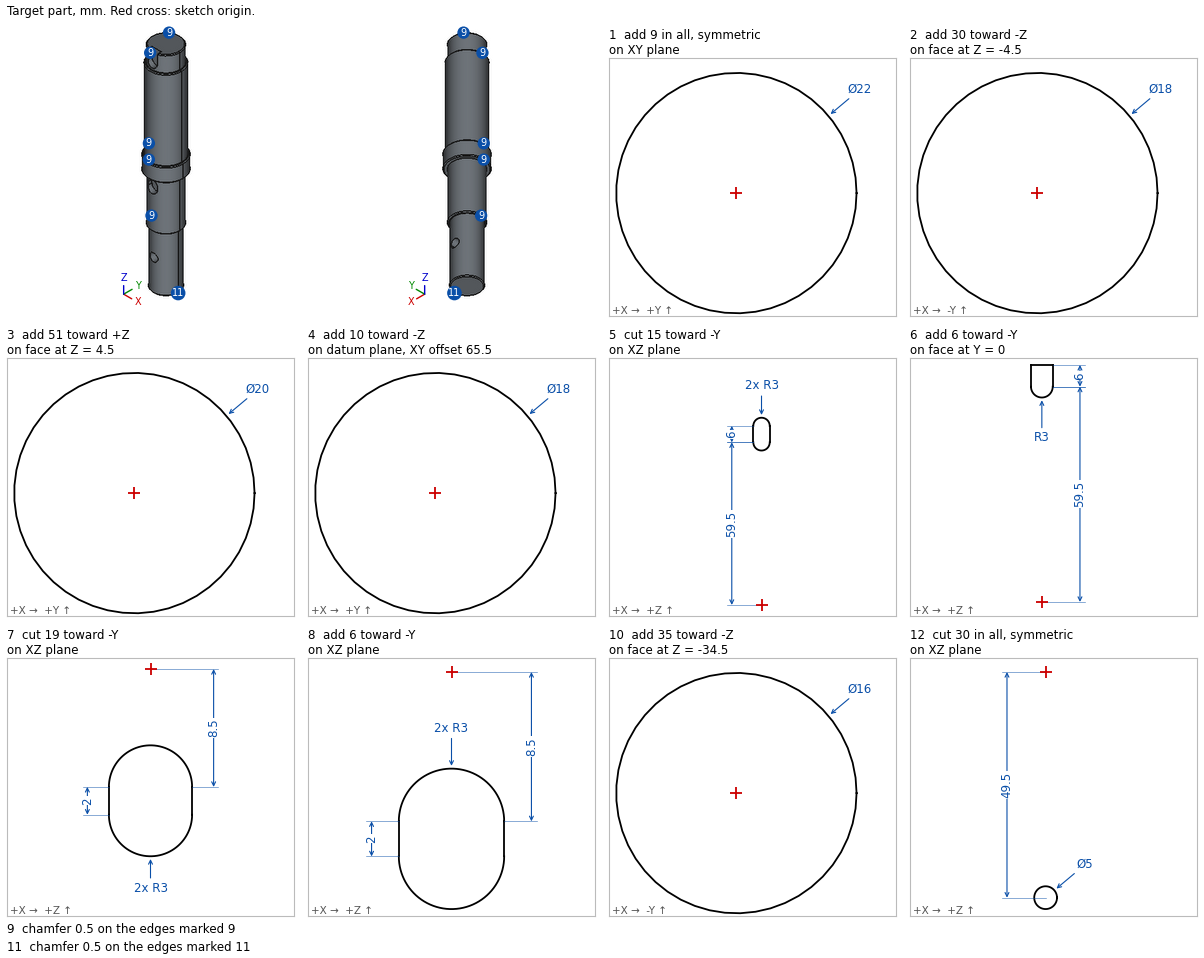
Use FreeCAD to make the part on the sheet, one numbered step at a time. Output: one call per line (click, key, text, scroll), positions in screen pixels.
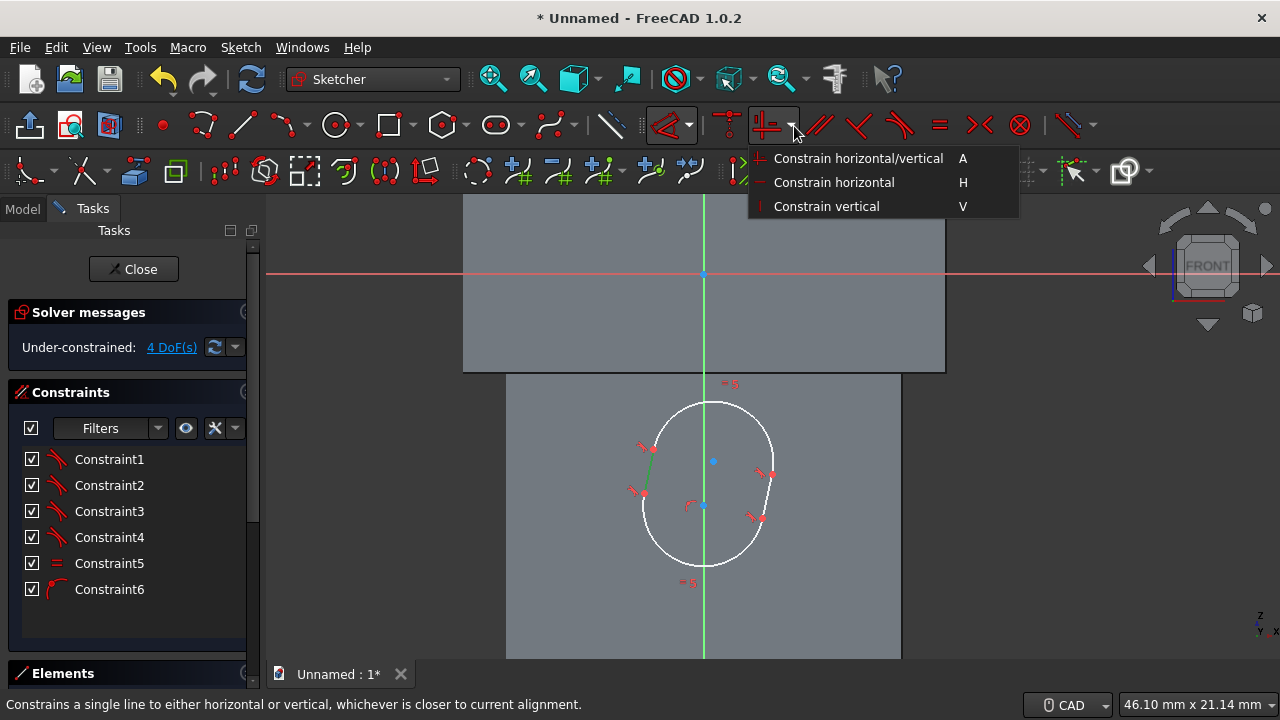
click(884, 206)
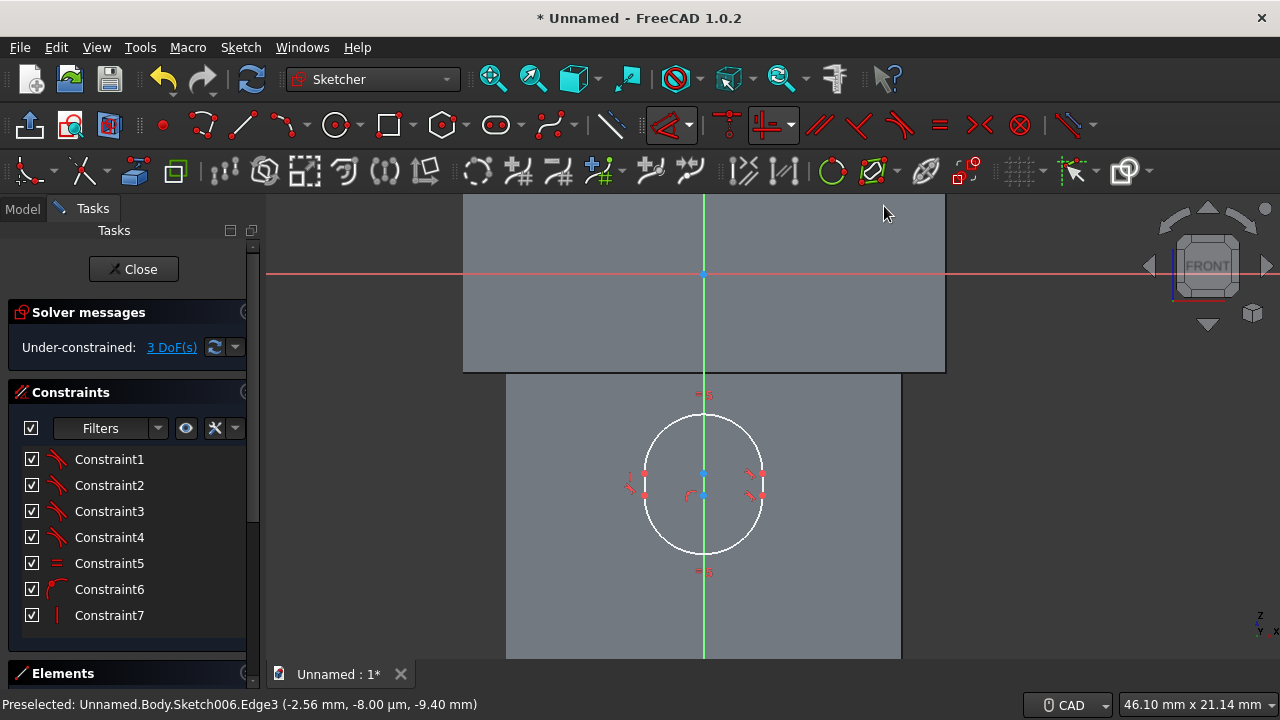
click(669, 543)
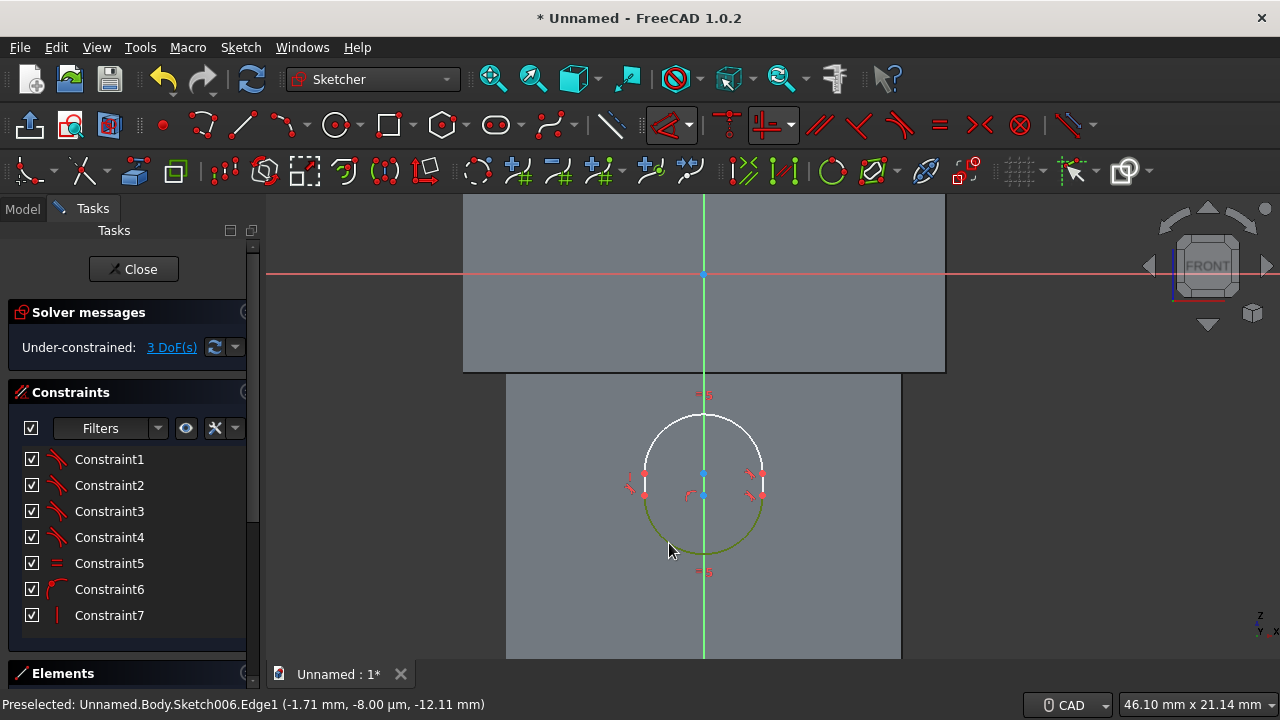
key(k)
key(r)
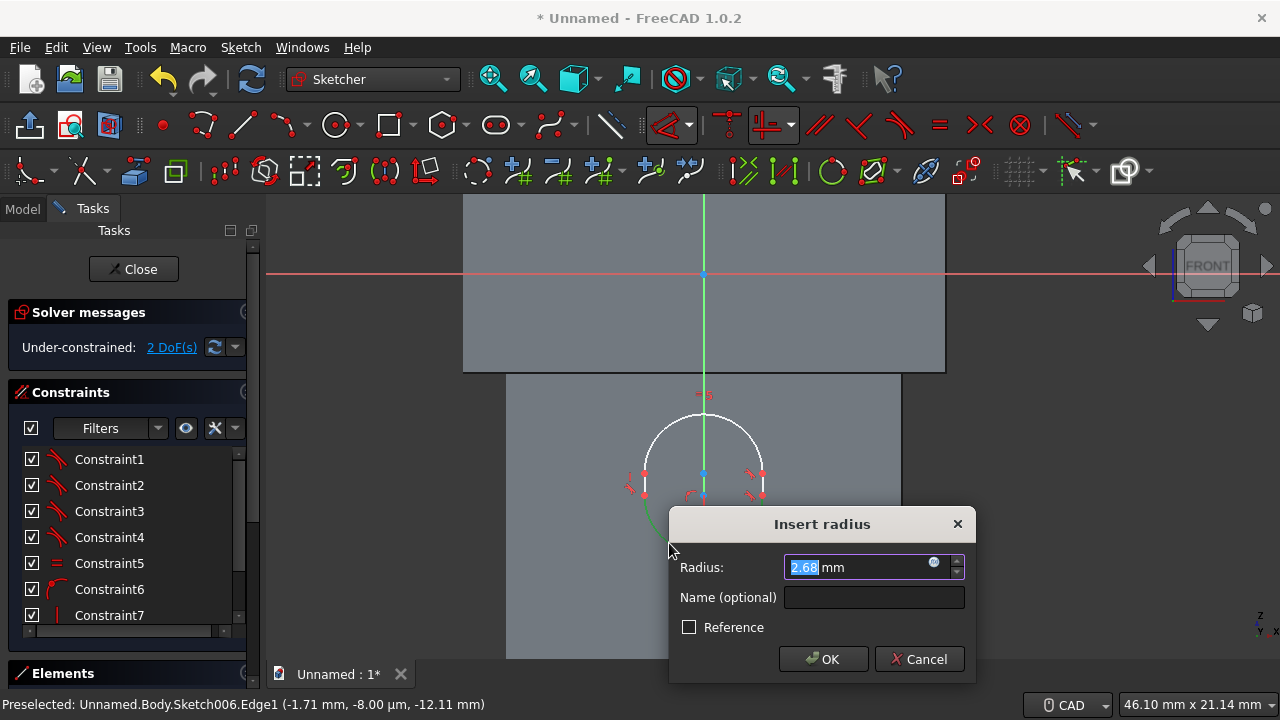
text(3)
key(Return)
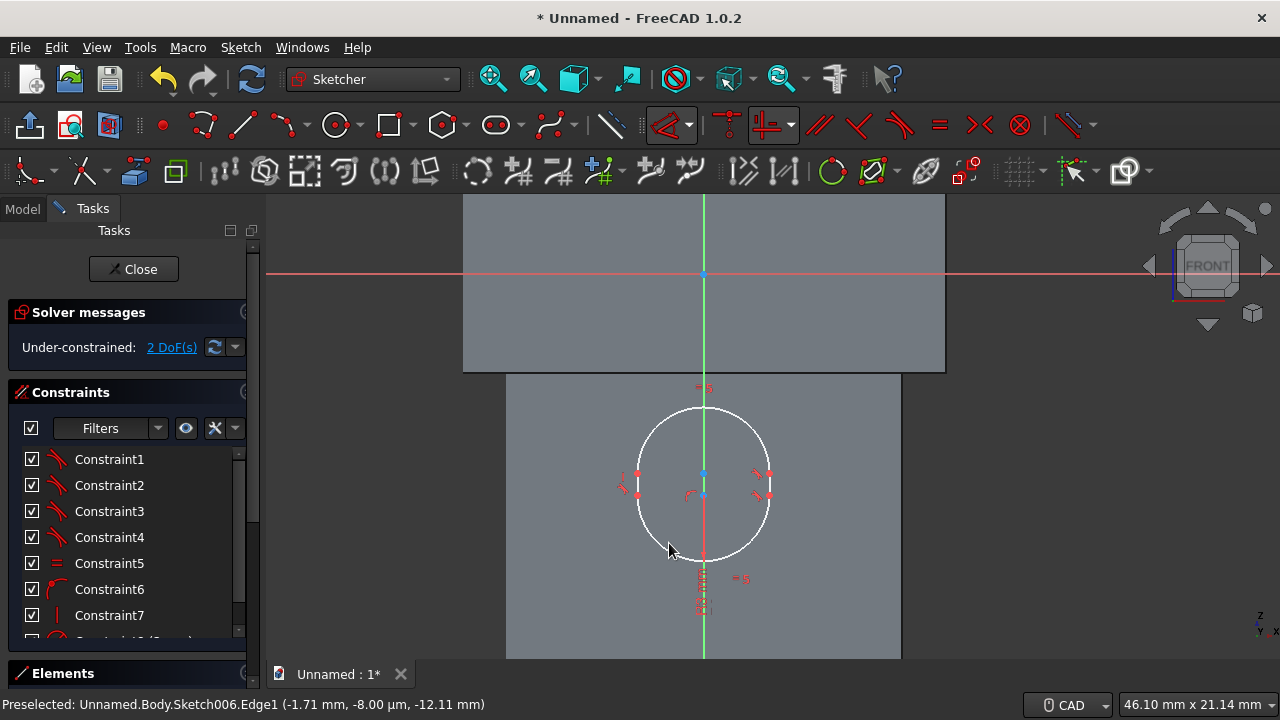
scroll(638, 484, up, 2)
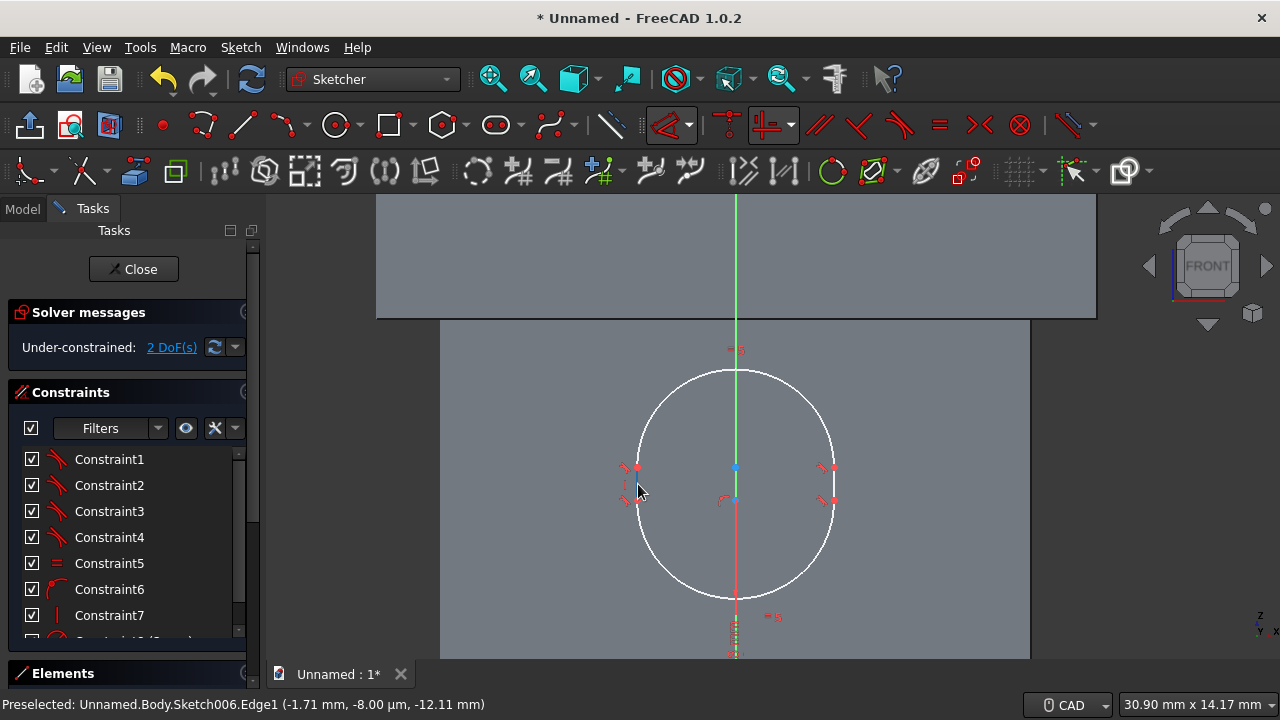
click(637, 484)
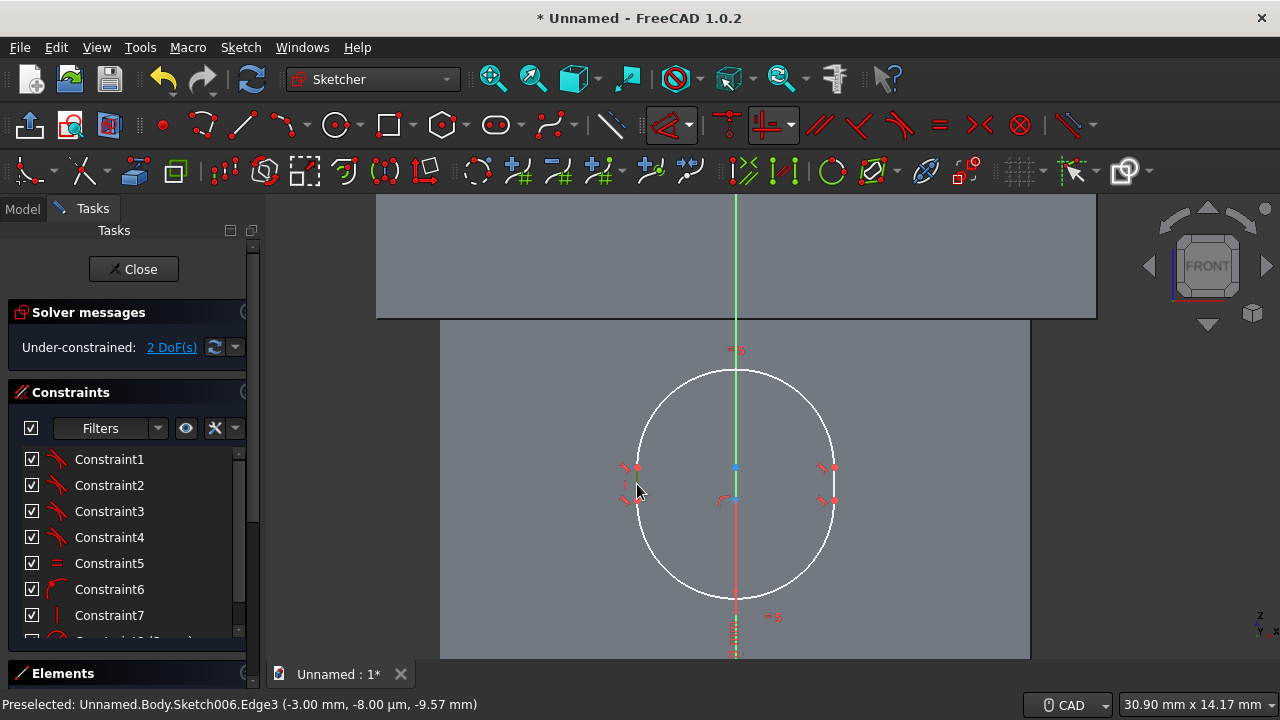
click(692, 126)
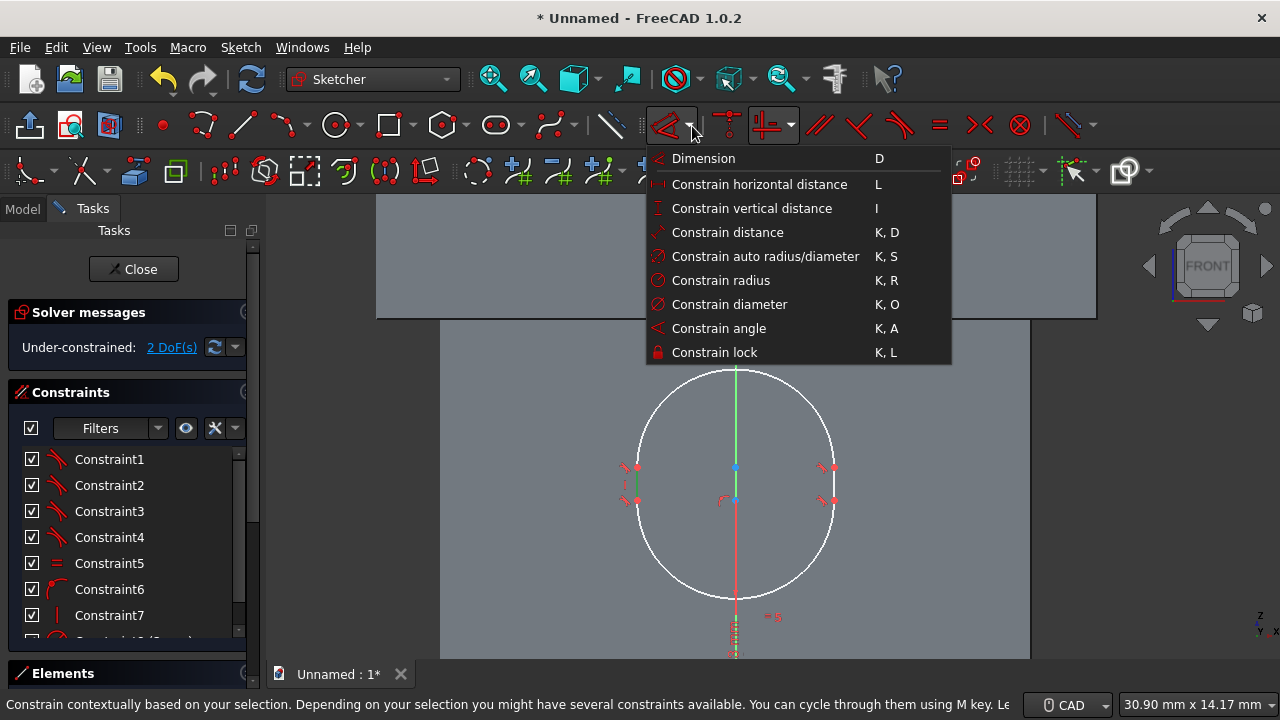
click(799, 208)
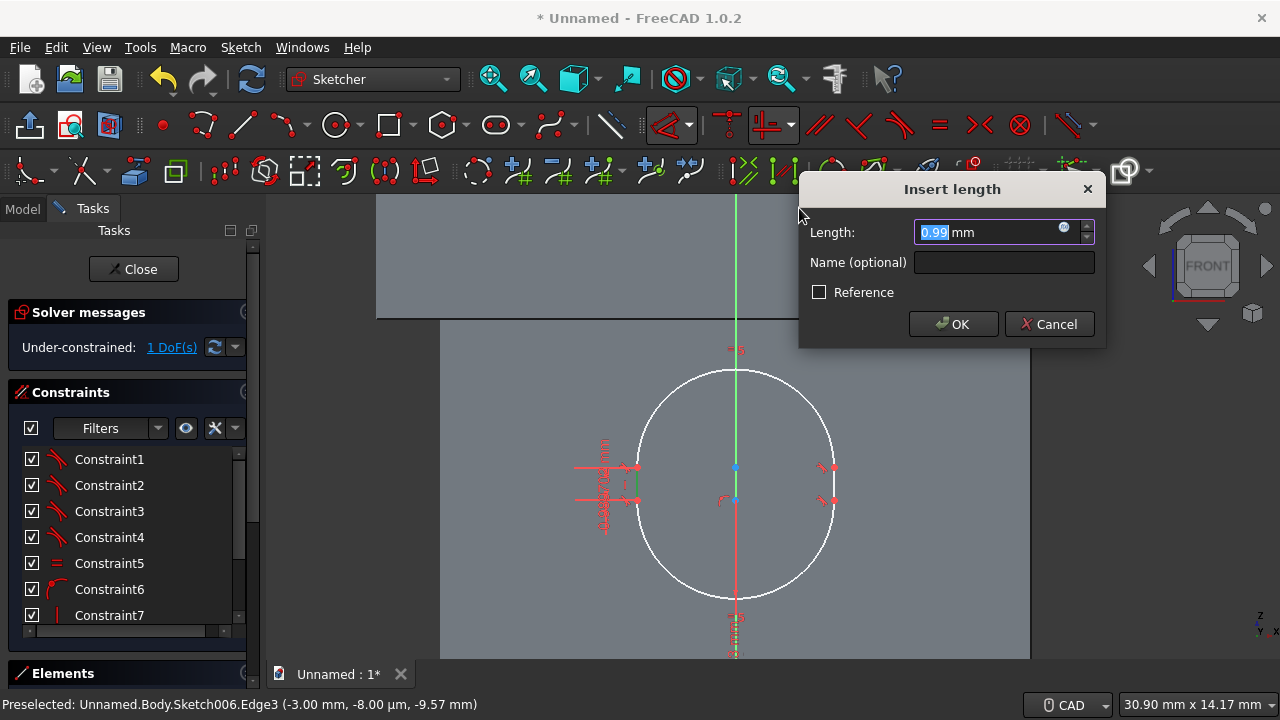
text(2)
key(Return)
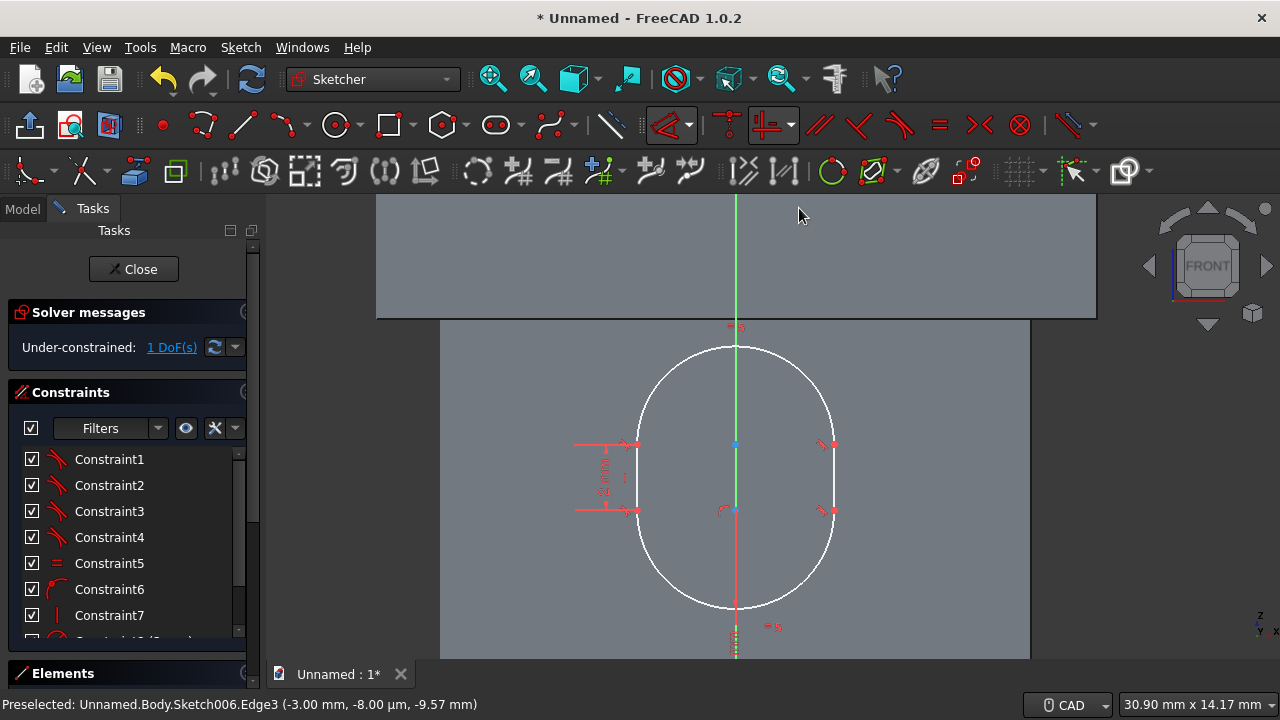
click(834, 445)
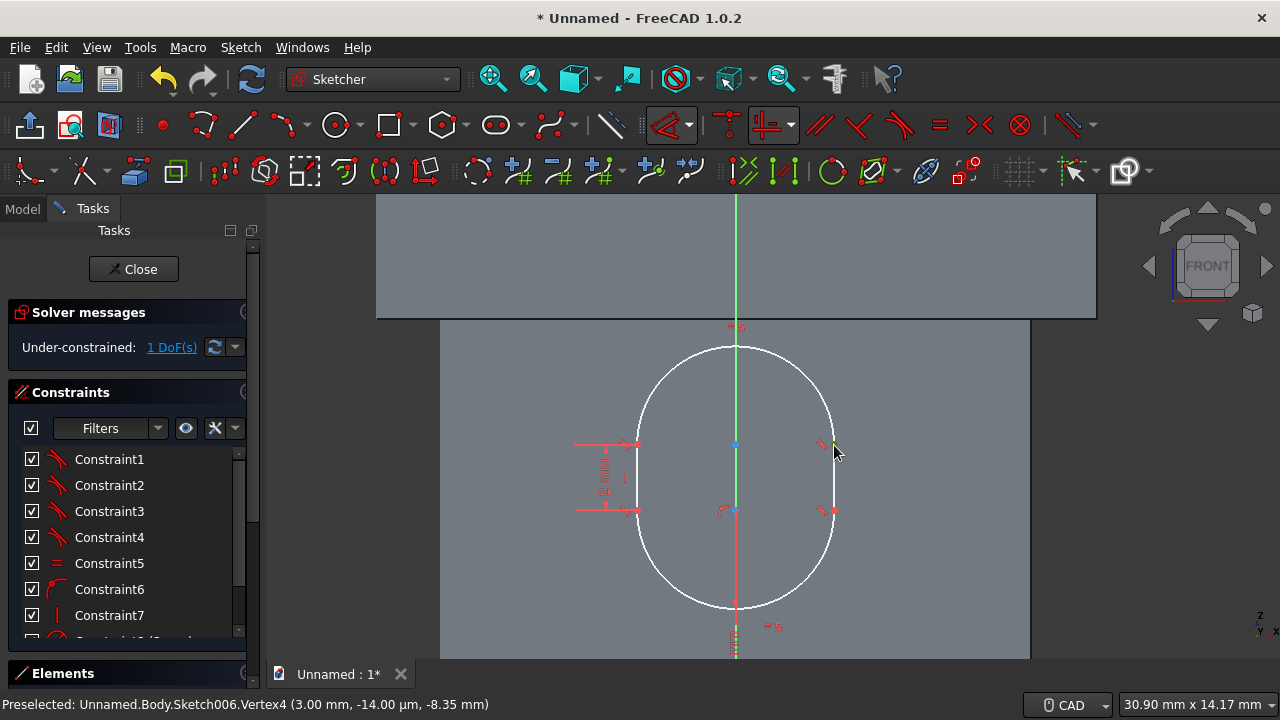
key(i)